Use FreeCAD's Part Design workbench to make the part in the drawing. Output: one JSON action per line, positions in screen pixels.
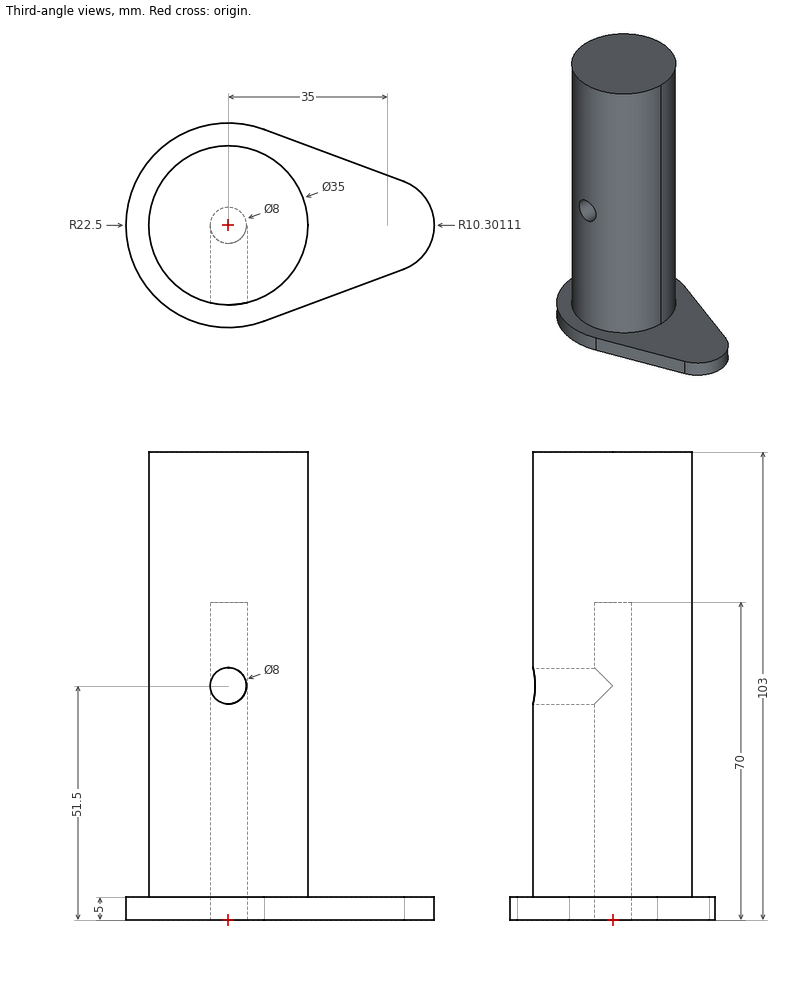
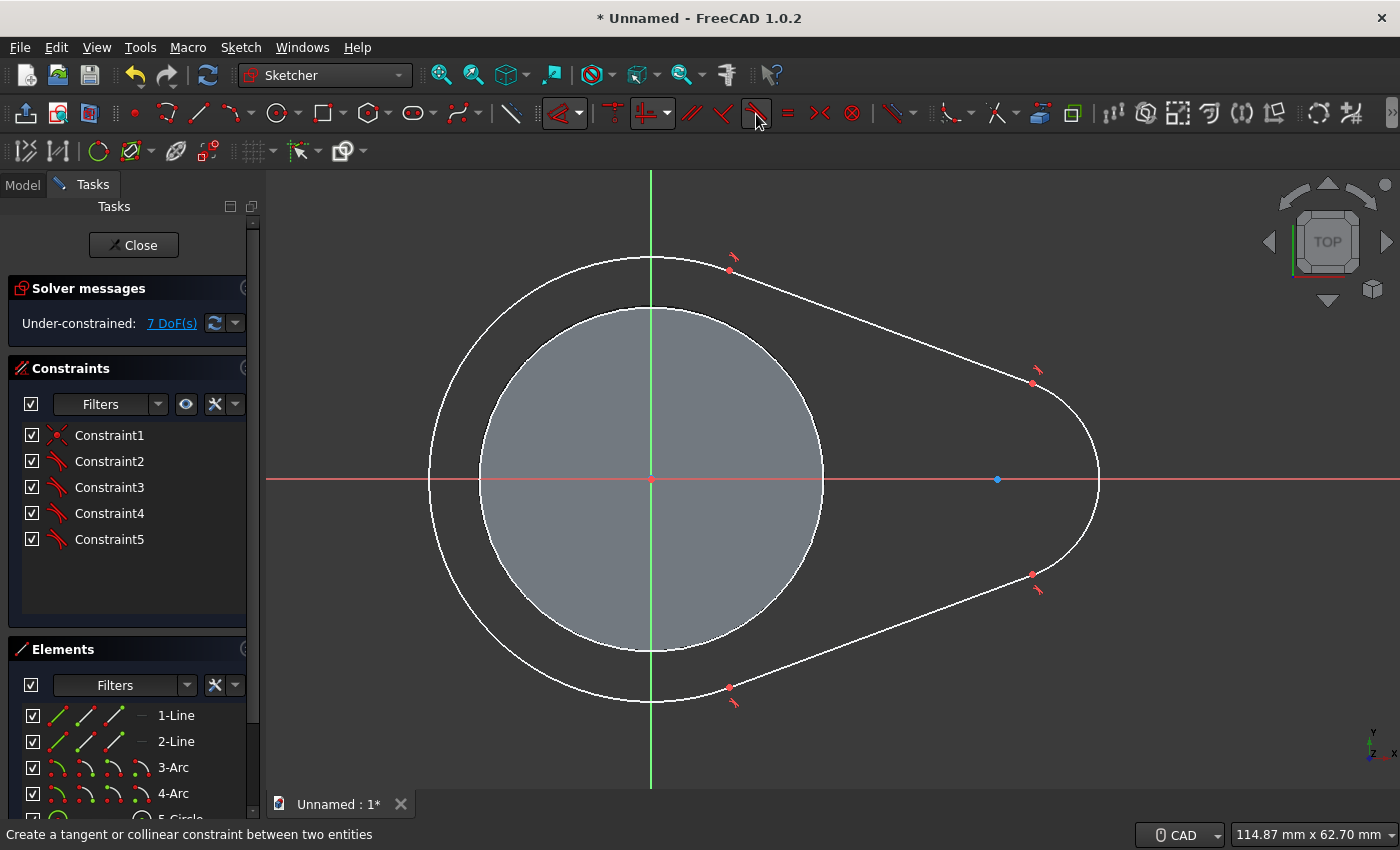
{"action": "left_click_drag", "start_coordinate": [641, 469], "coordinate": [661, 490]}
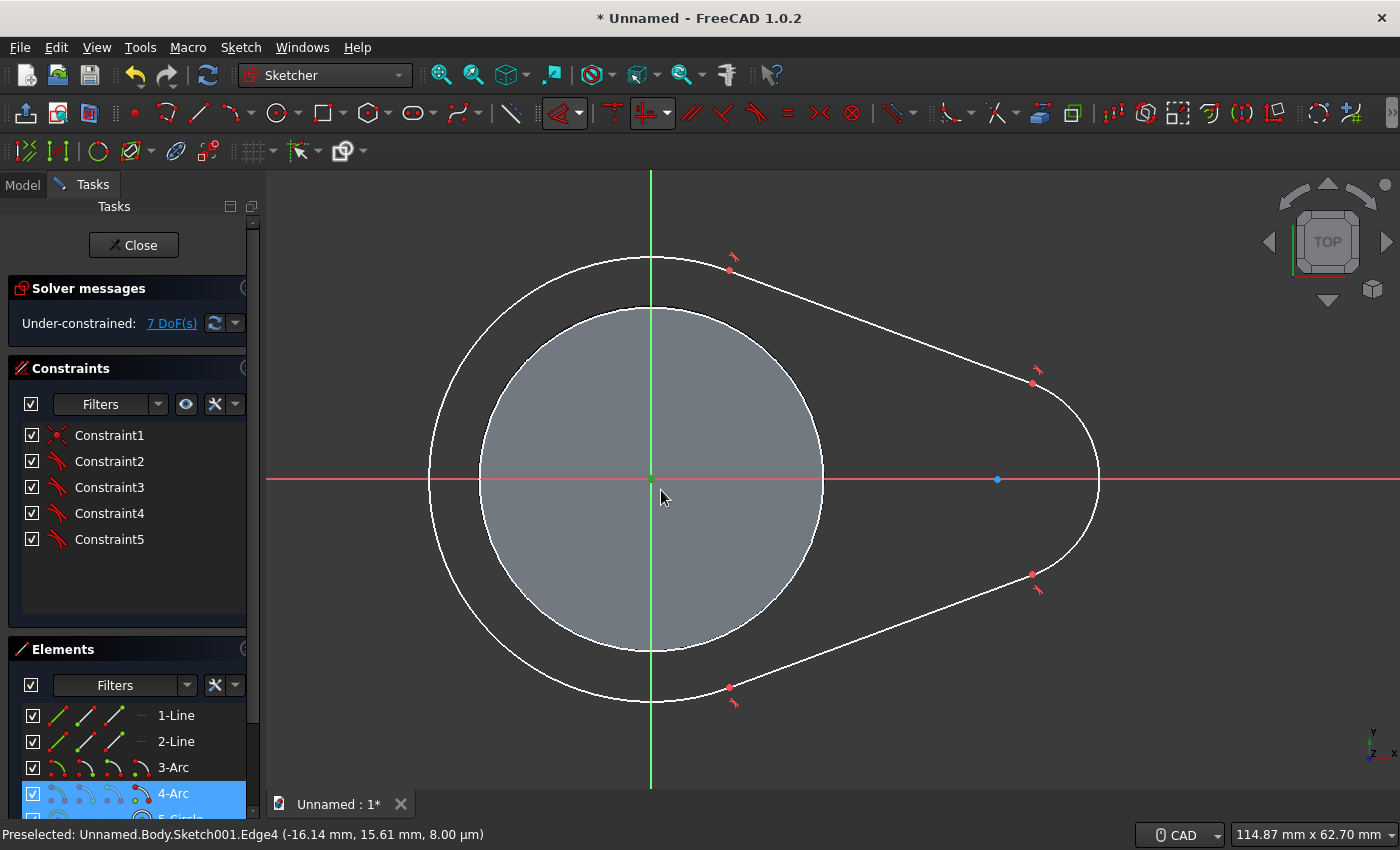
{"action": "left_click", "coordinate": [614, 114]}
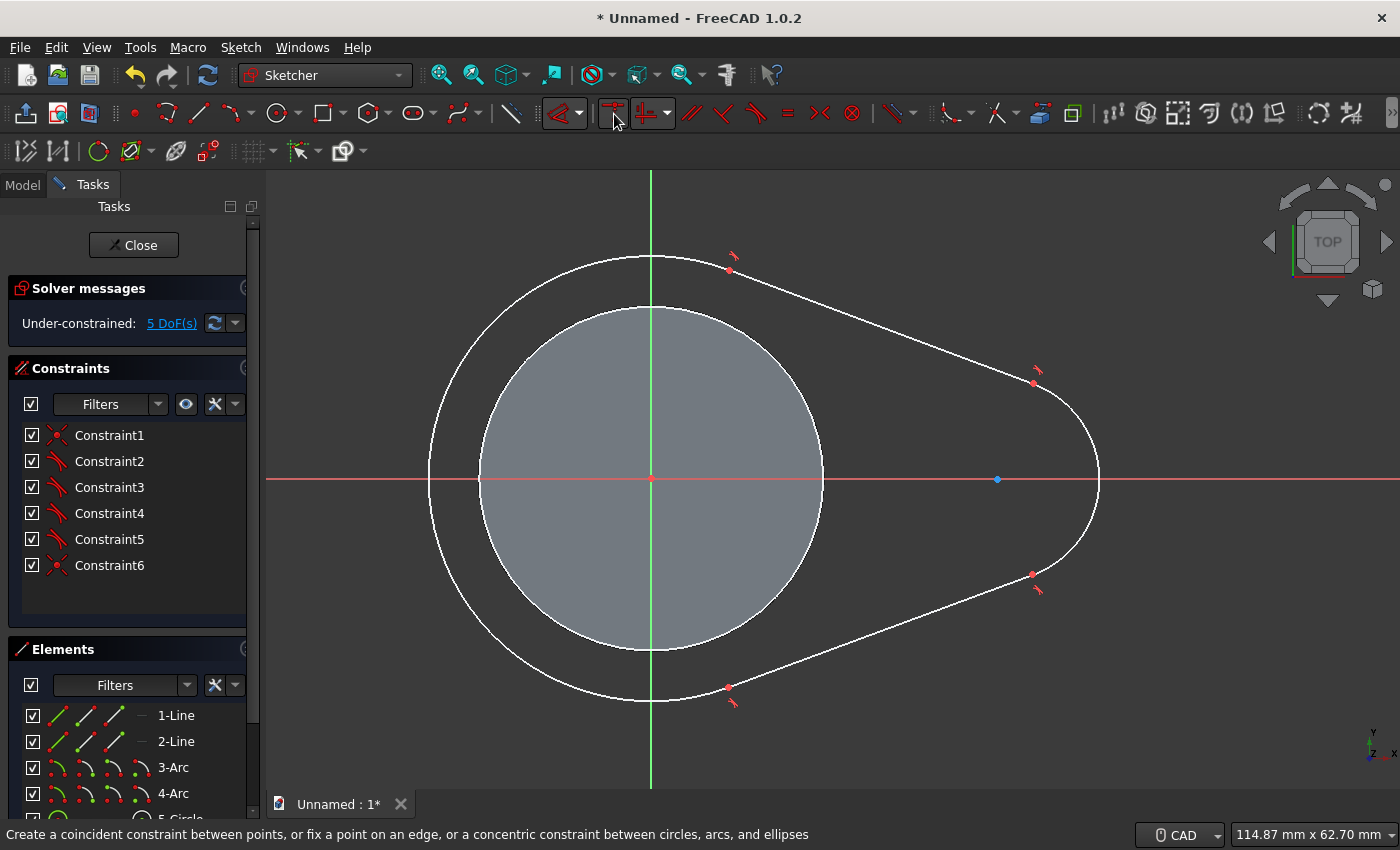
{"action": "left_click", "coordinate": [997, 479]}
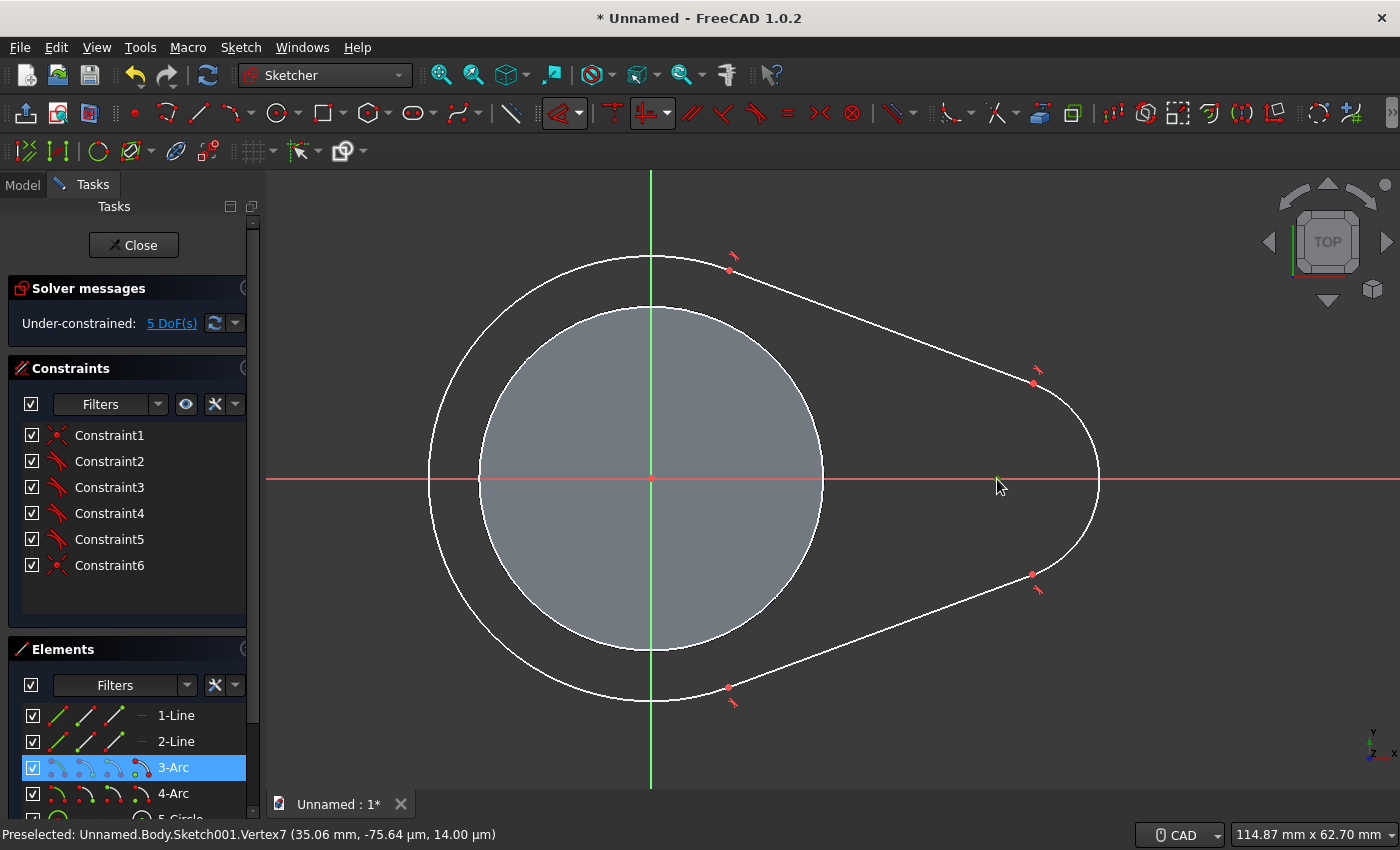
{"action": "left_click", "coordinate": [361, 479]}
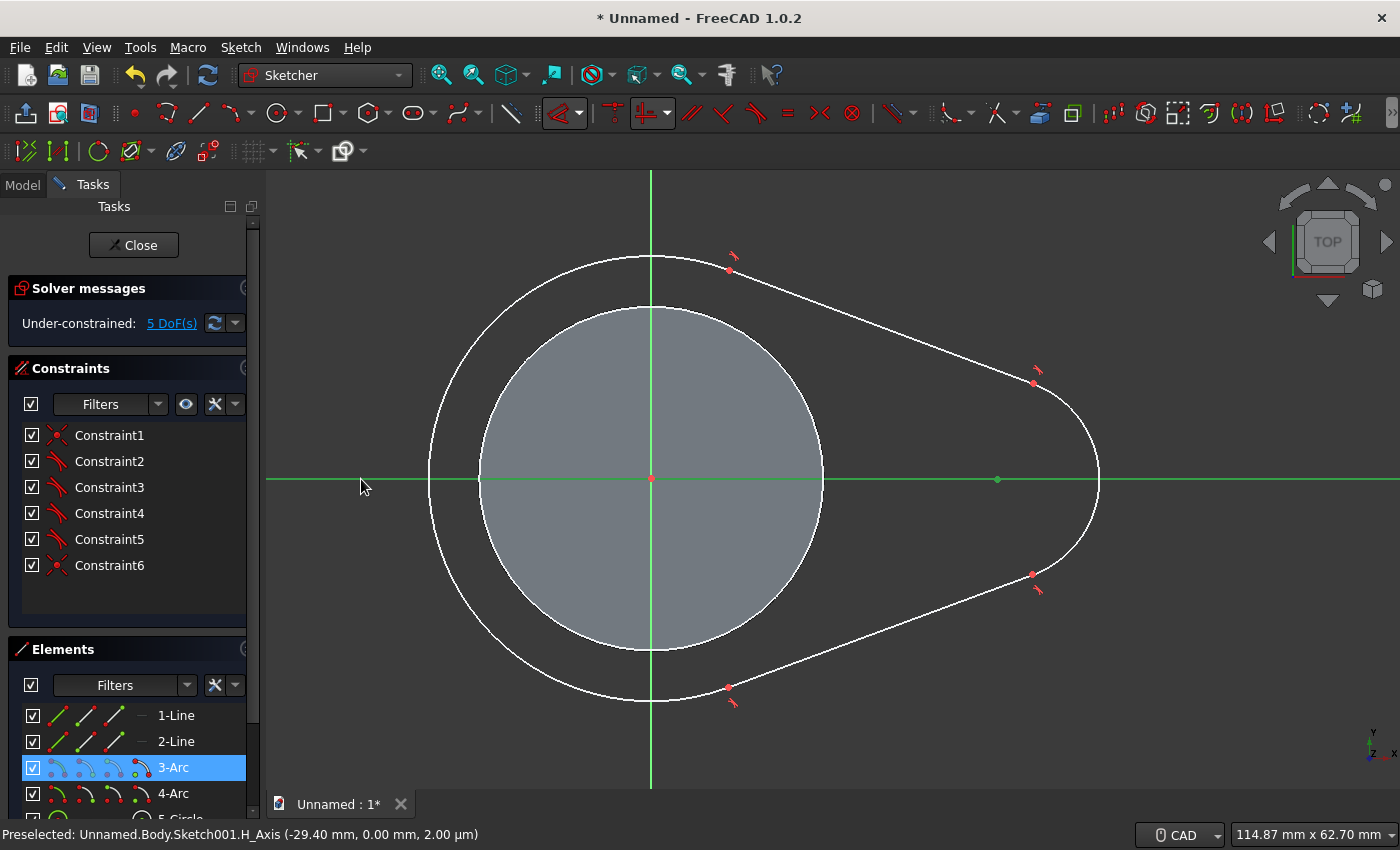
{"action": "left_click", "coordinate": [614, 114]}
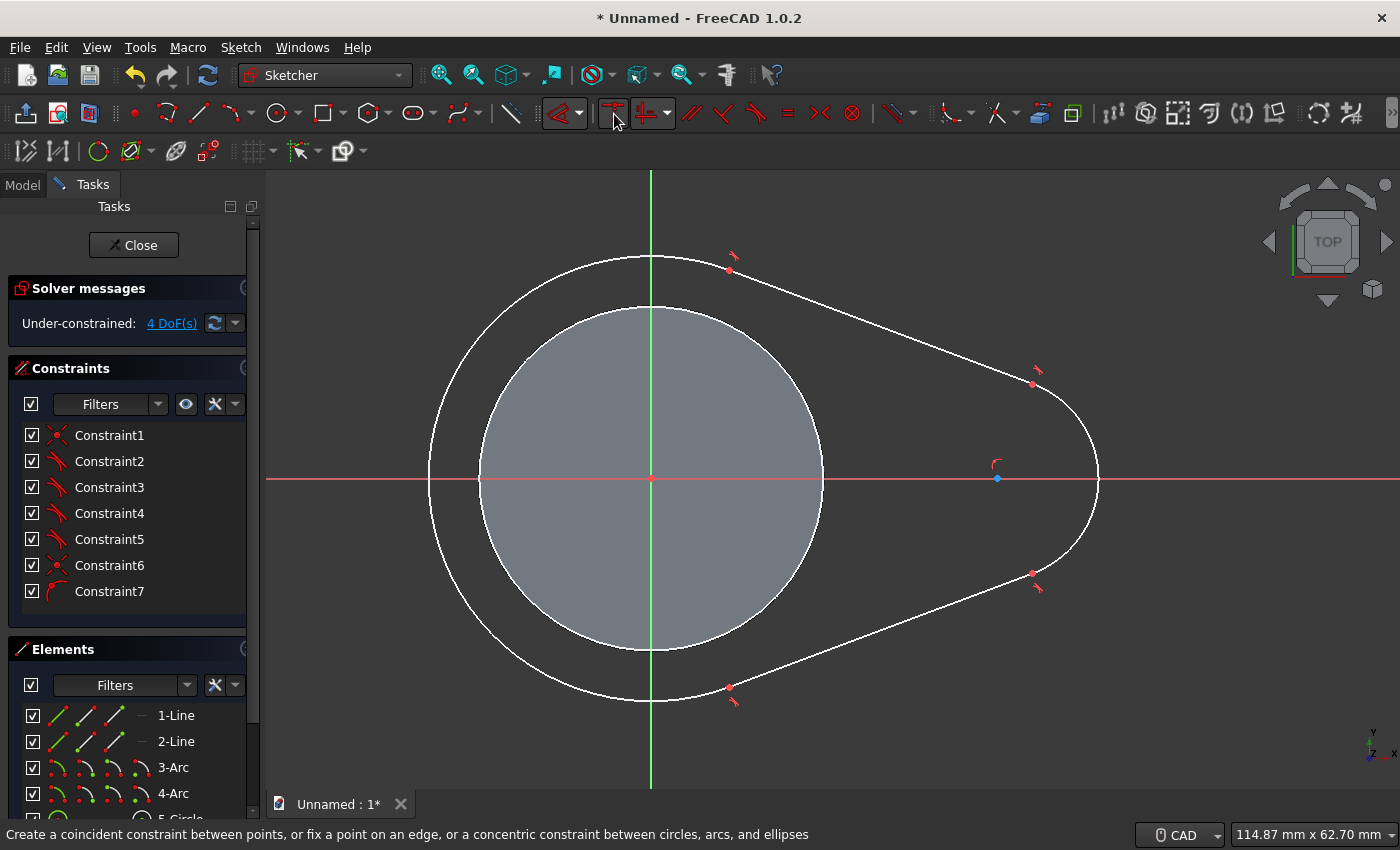
{"action": "left_click", "coordinate": [1087, 526]}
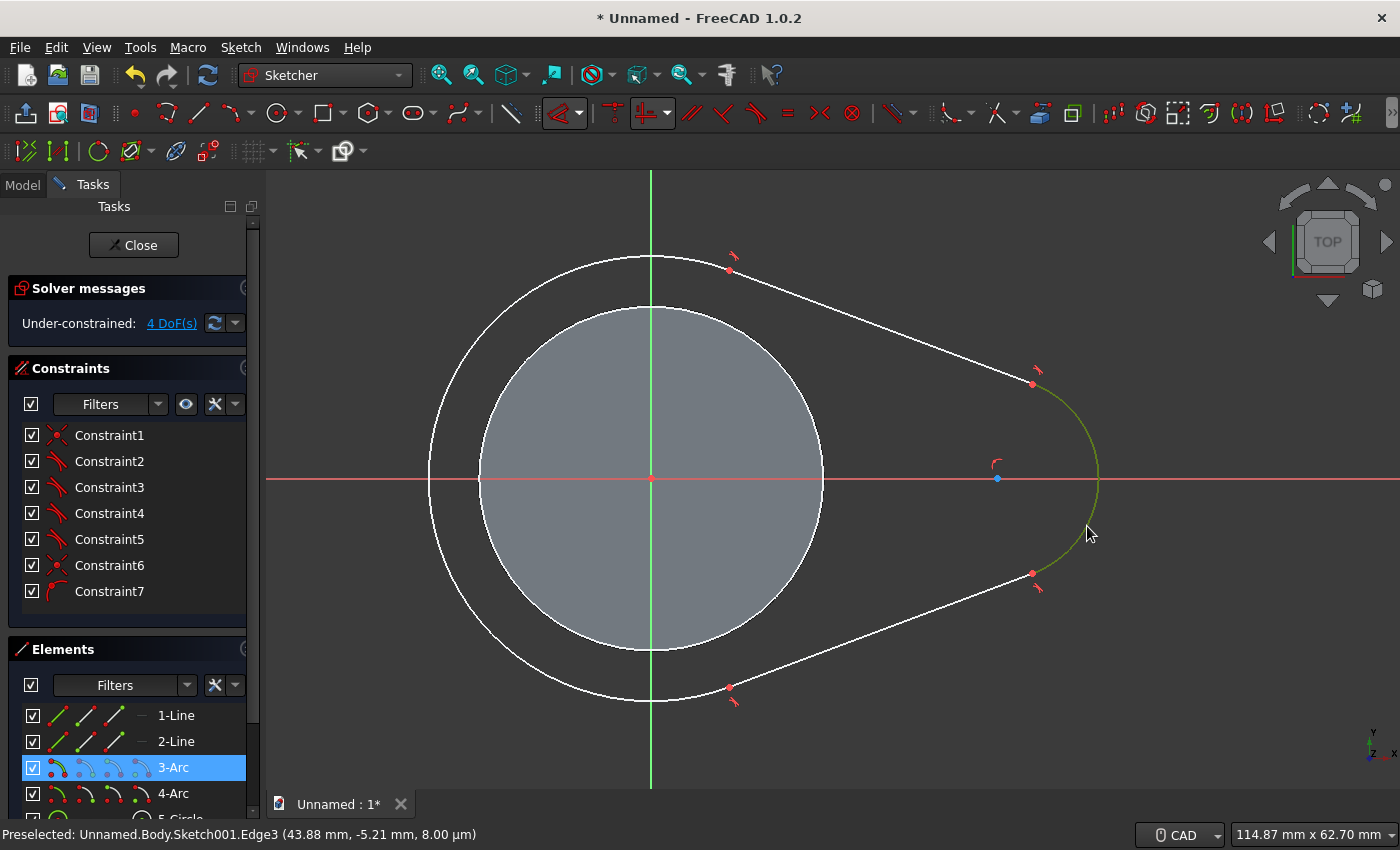
{"action": "key", "text": "k r"}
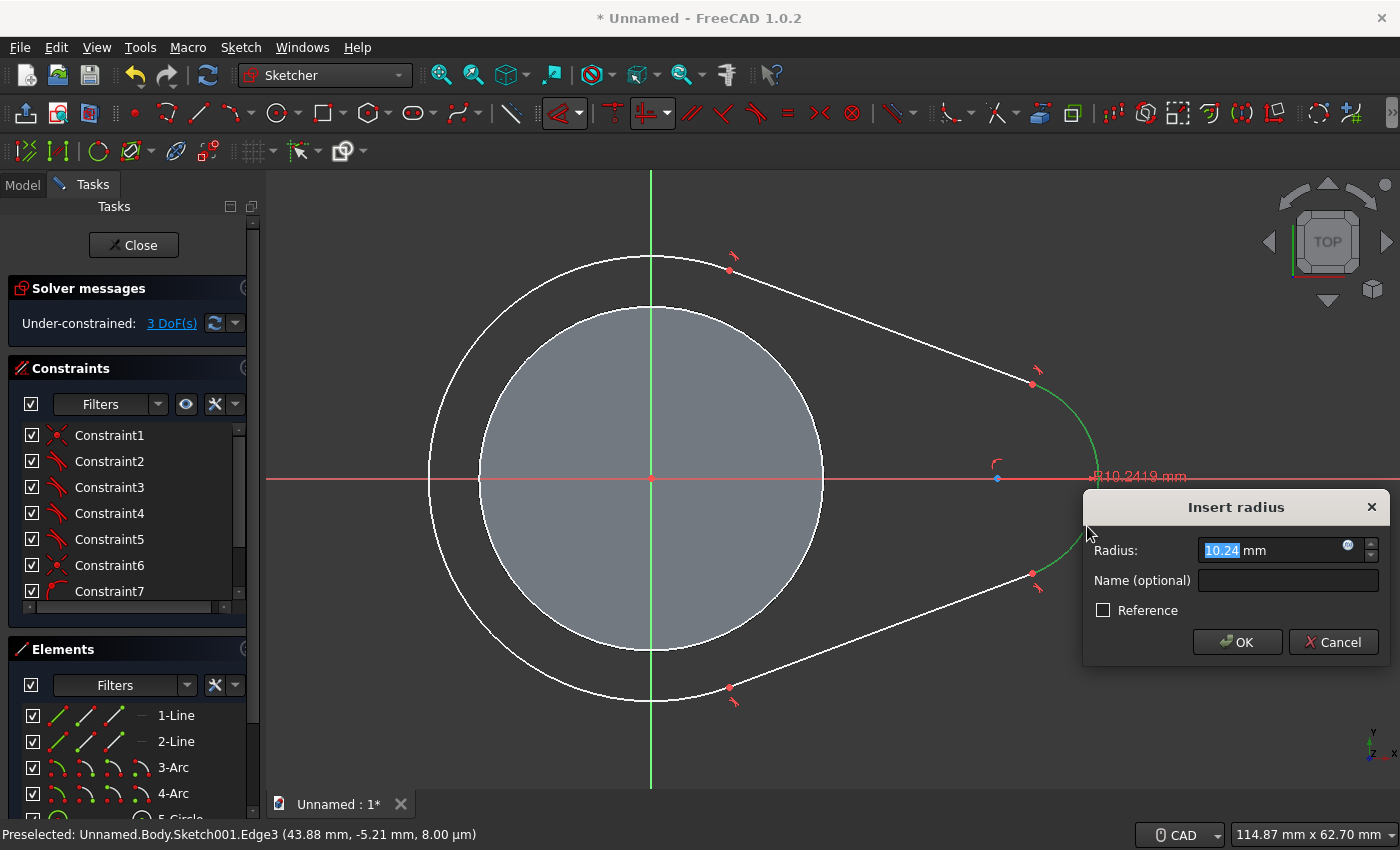
{"action": "type", "text": "10.30111"}
{"action": "key", "text": "Return"}